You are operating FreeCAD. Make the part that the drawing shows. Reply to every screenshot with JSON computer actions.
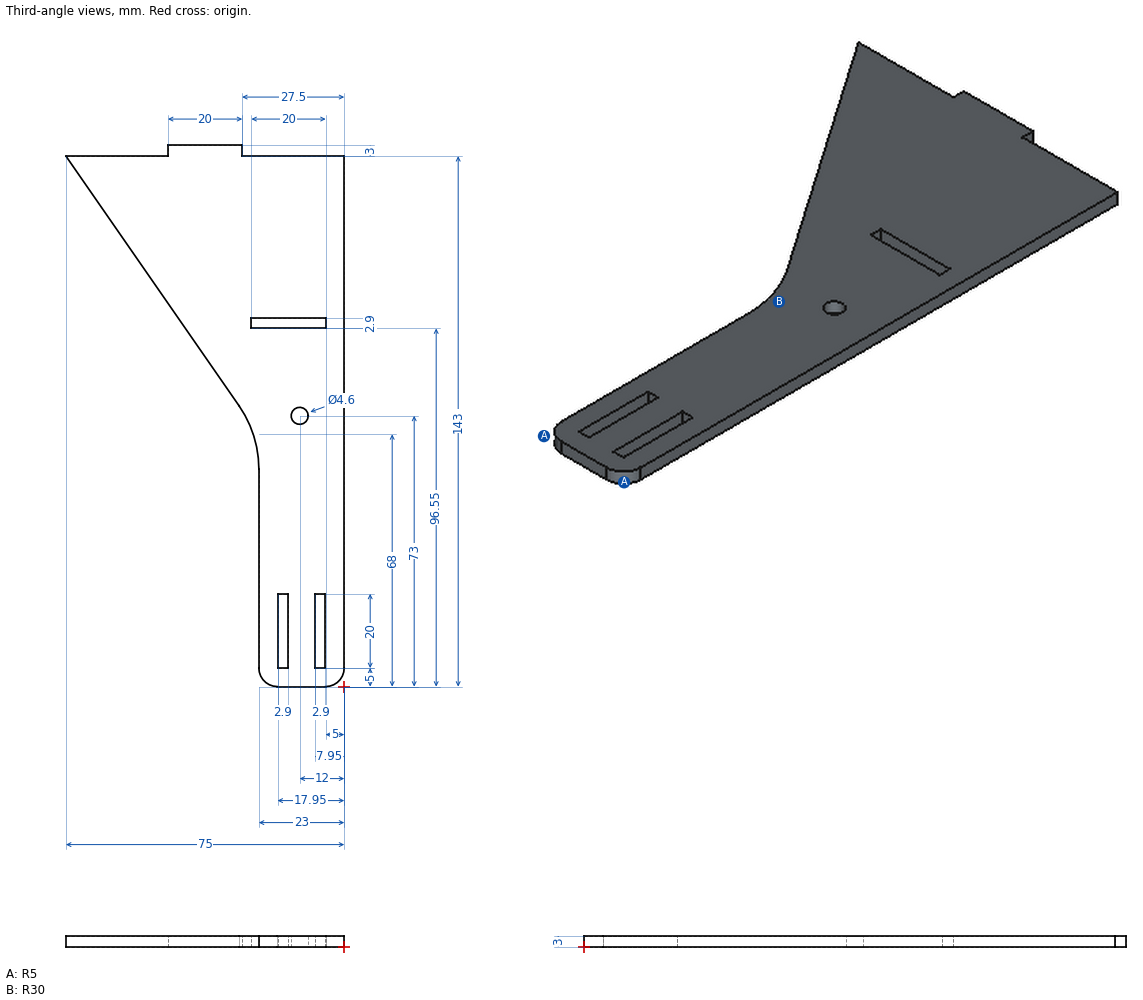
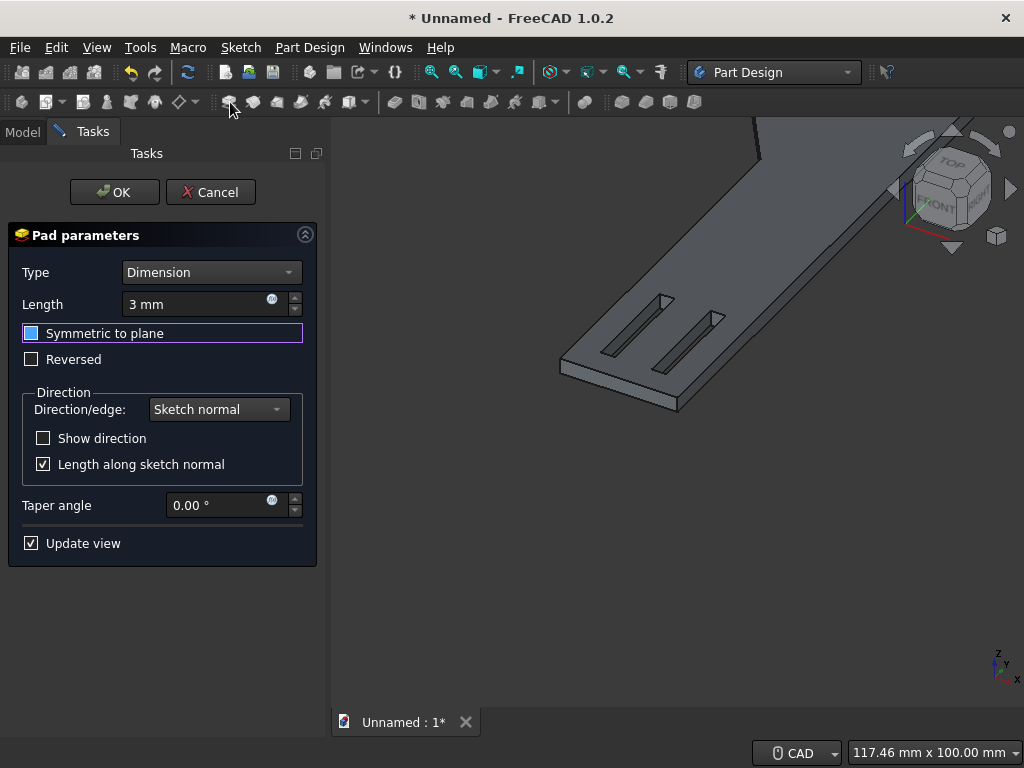
{"action": "left_click", "coordinate": [115, 192]}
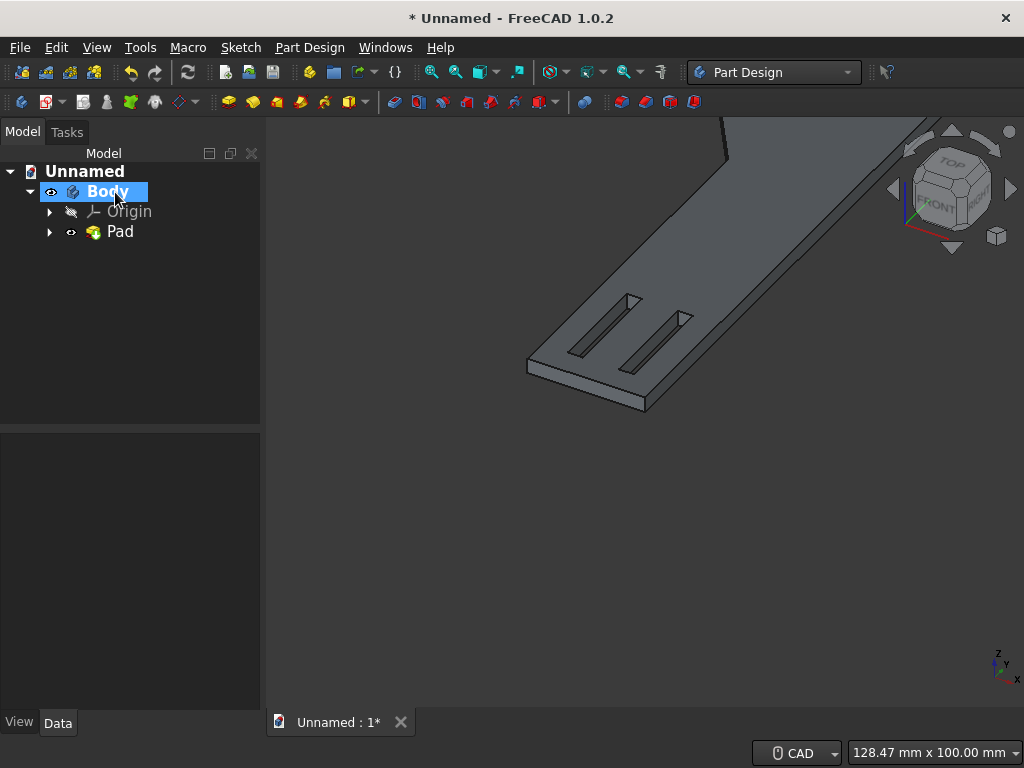
{"action": "left_click", "coordinate": [432, 72]}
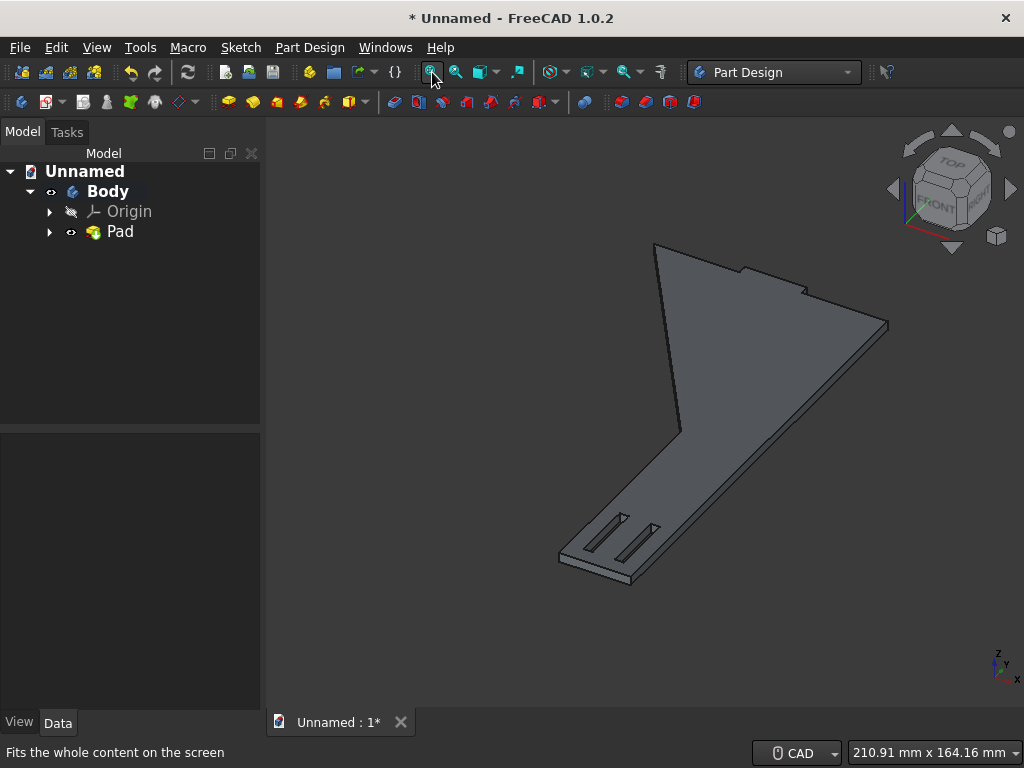
{"action": "left_click", "coordinate": [631, 582]}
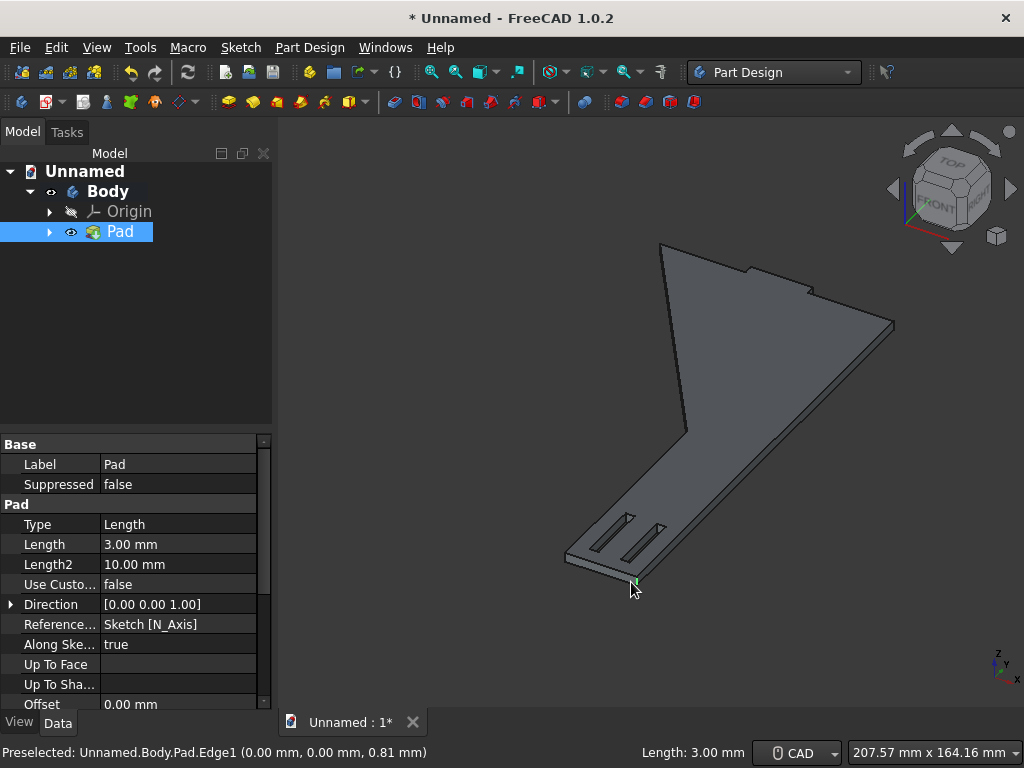
{"action": "scroll", "coordinate": [565, 556], "scroll_direction": "up", "scroll_amount": 7}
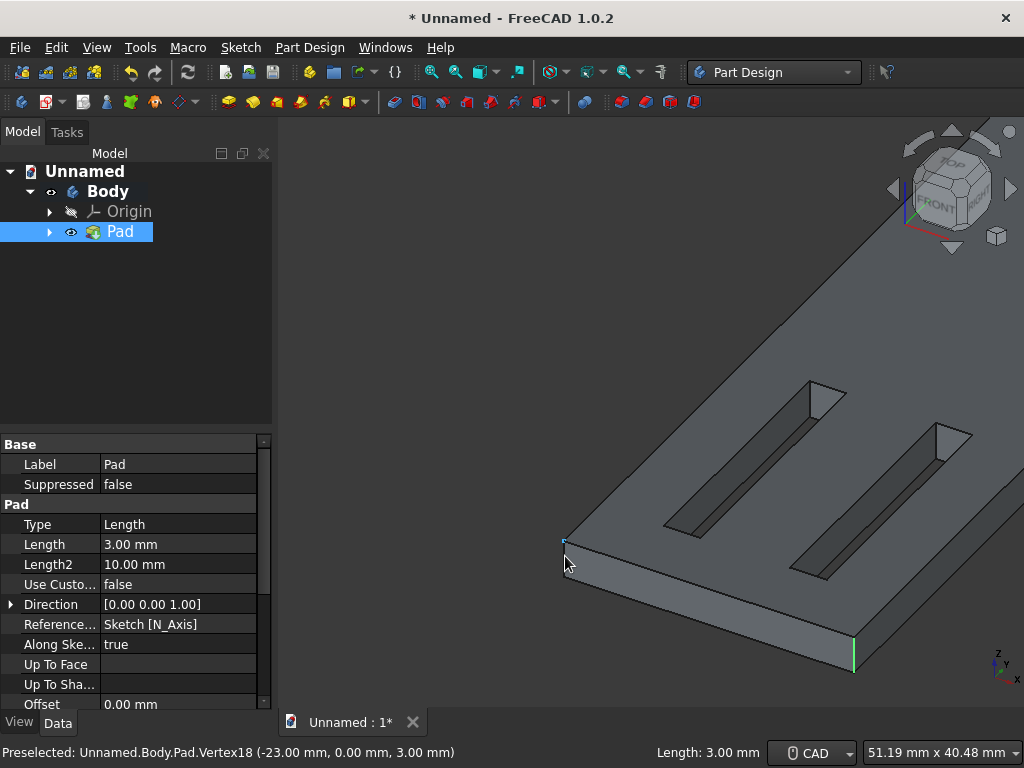
{"action": "left_click", "coordinate": [432, 72]}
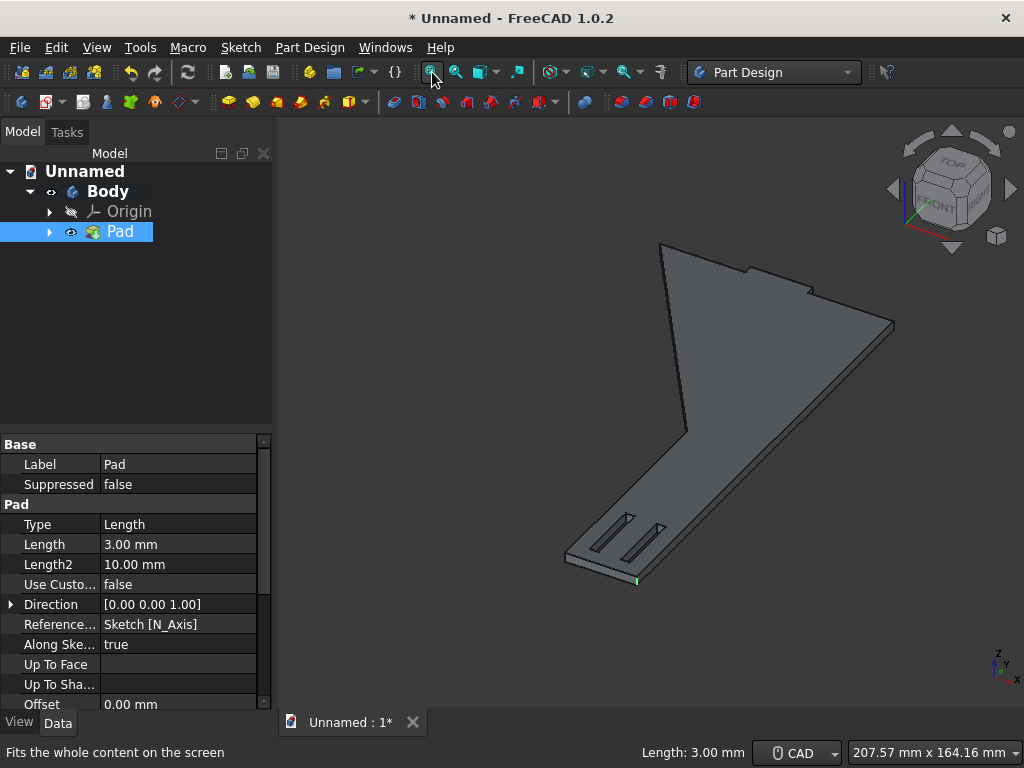
{"action": "key", "text": "0"}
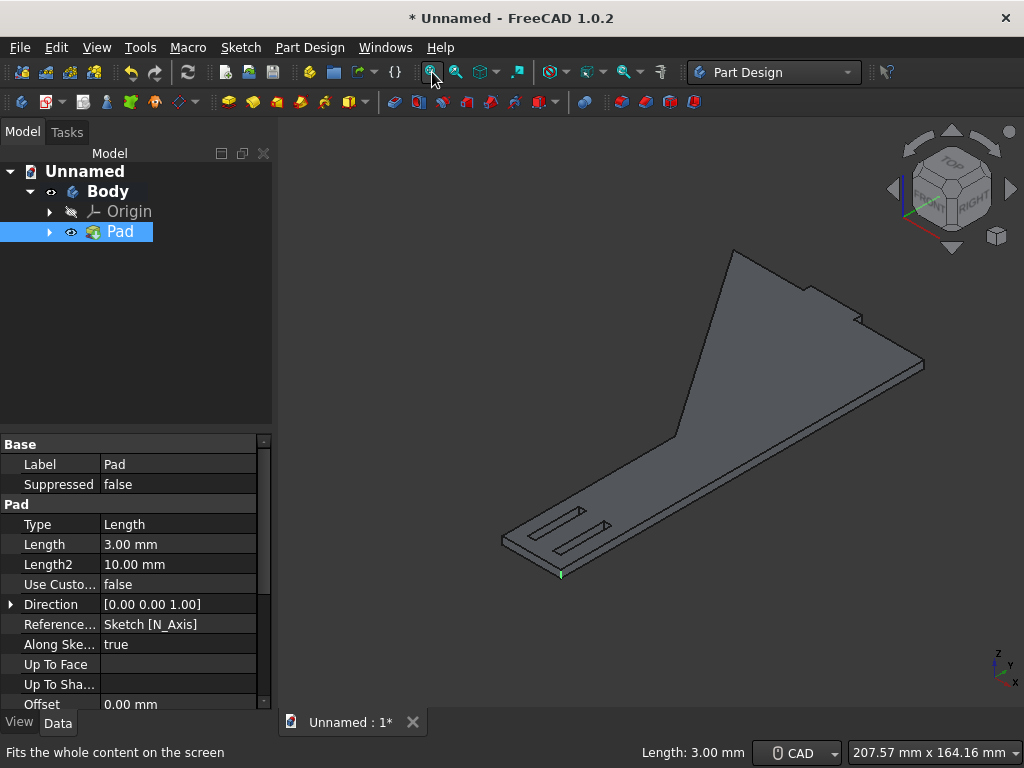
{"action": "scroll", "coordinate": [502, 539], "scroll_direction": "up", "scroll_amount": 7}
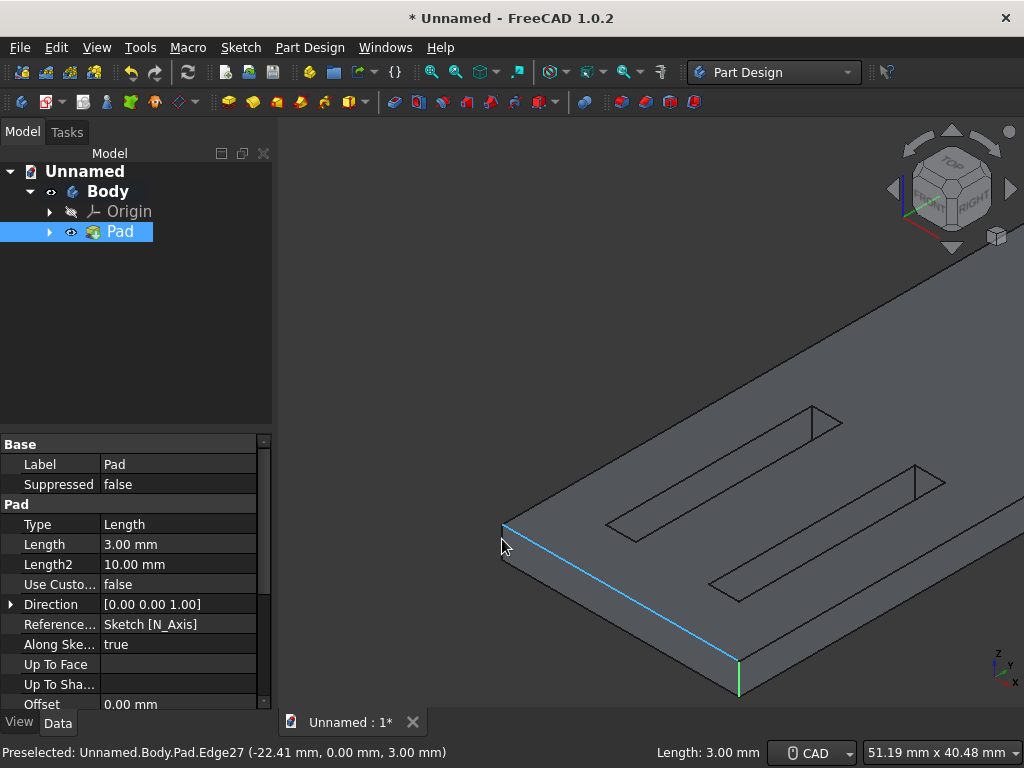
{"action": "left_click", "coordinate": [432, 72]}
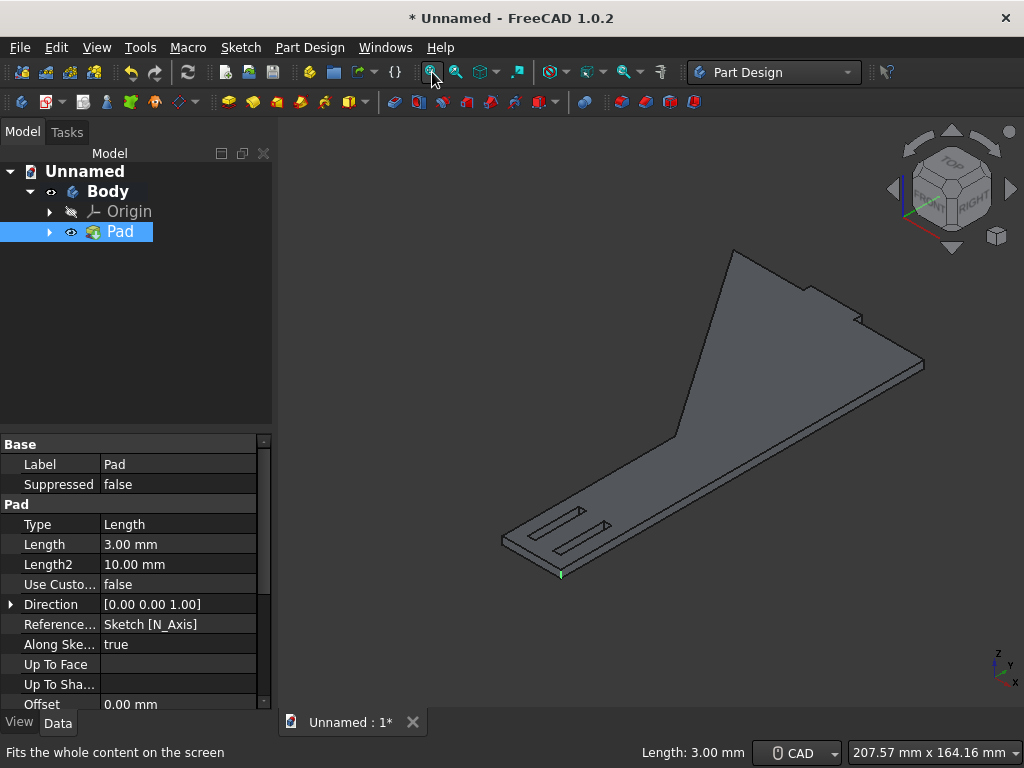
{"action": "key", "text": "2"}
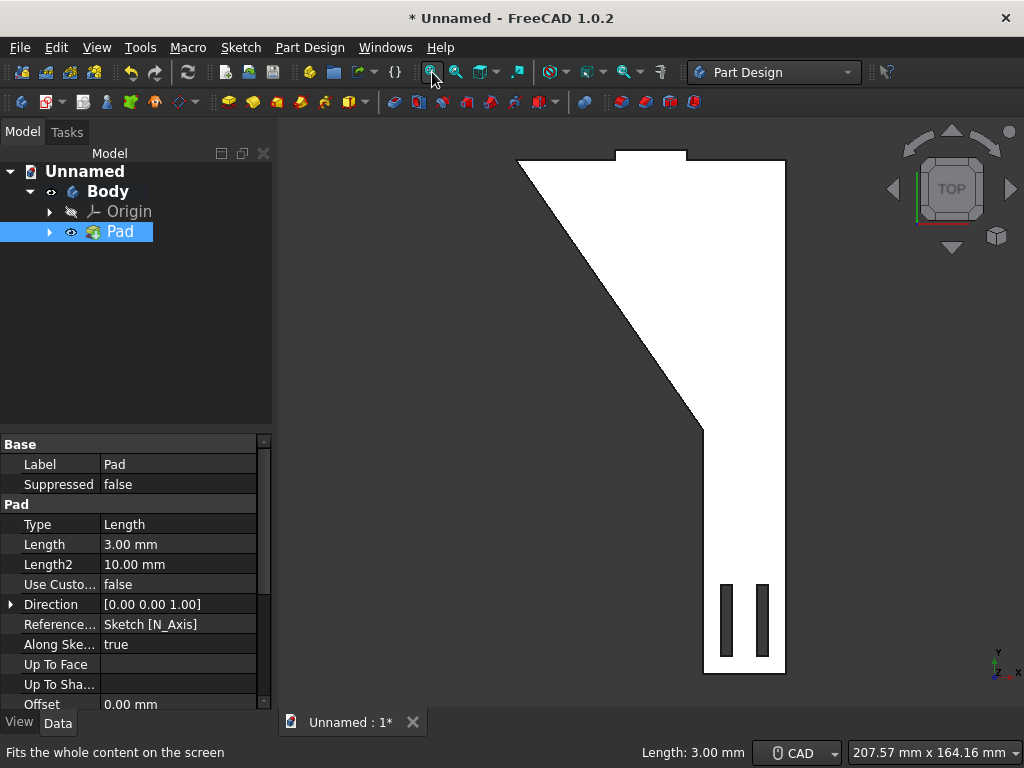
{"action": "scroll", "coordinate": [703, 673], "scroll_direction": "up", "scroll_amount": 7}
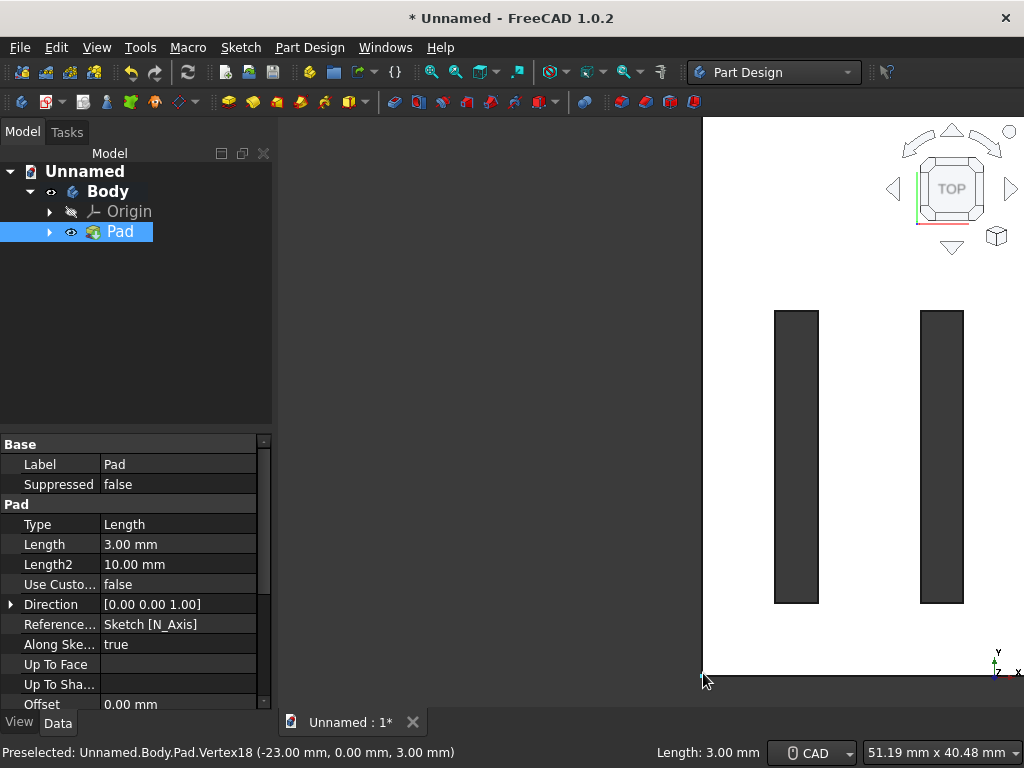
{"action": "left_click", "coordinate": [432, 72]}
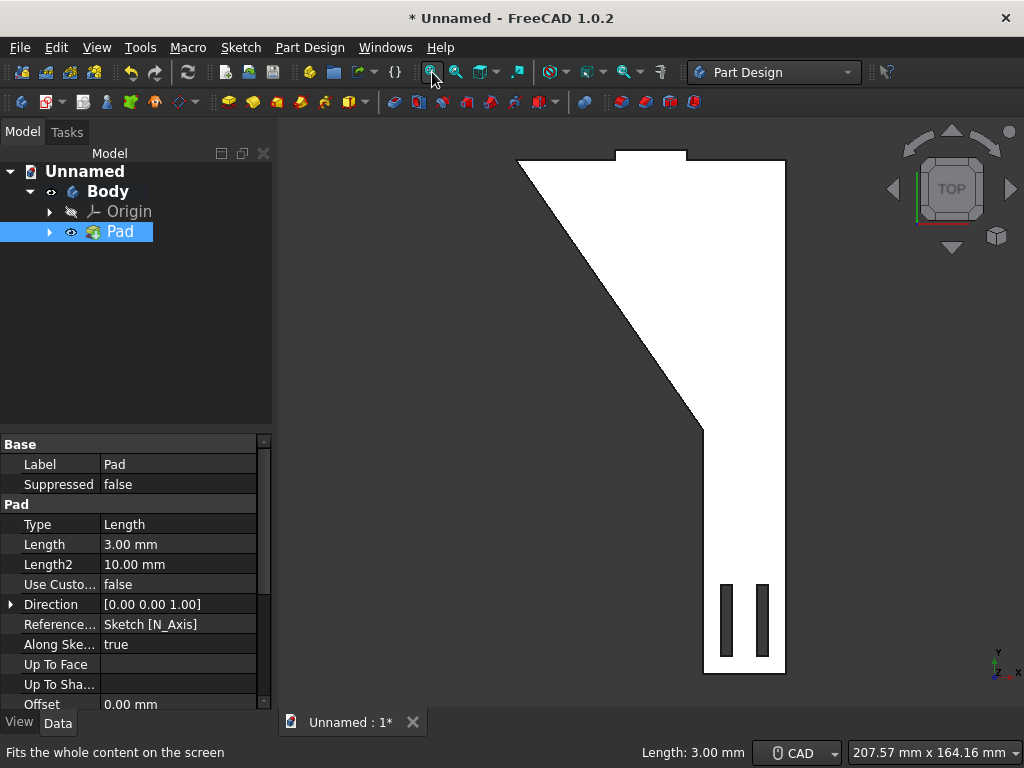
{"action": "key", "text": "1"}